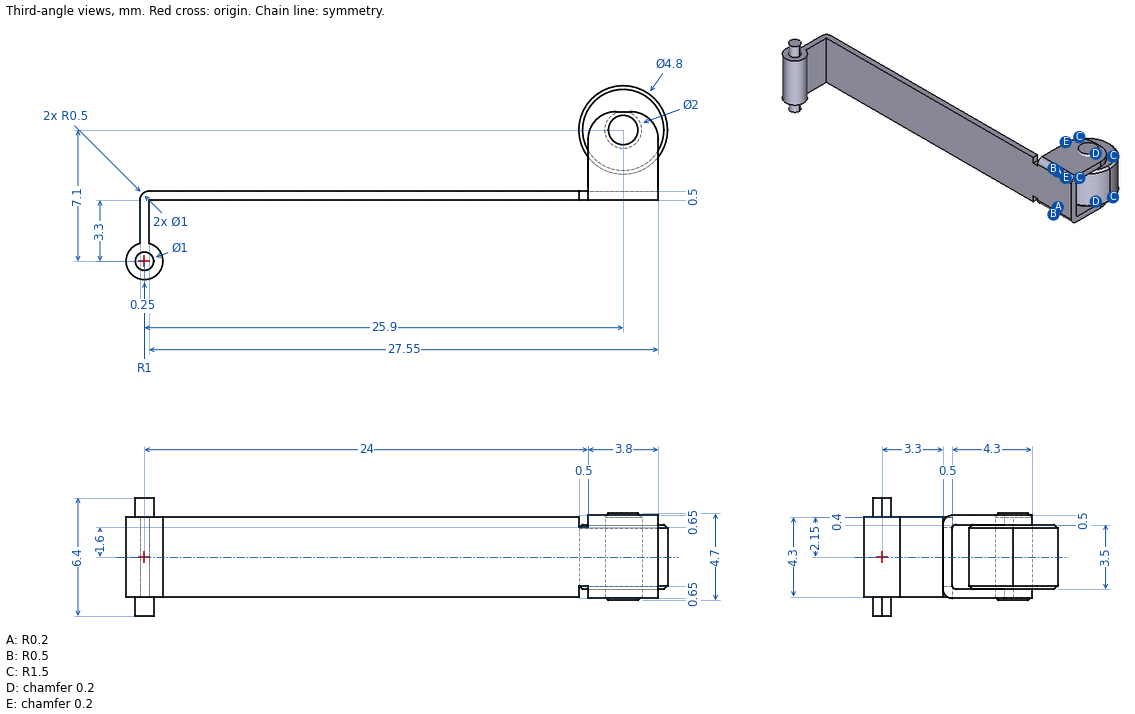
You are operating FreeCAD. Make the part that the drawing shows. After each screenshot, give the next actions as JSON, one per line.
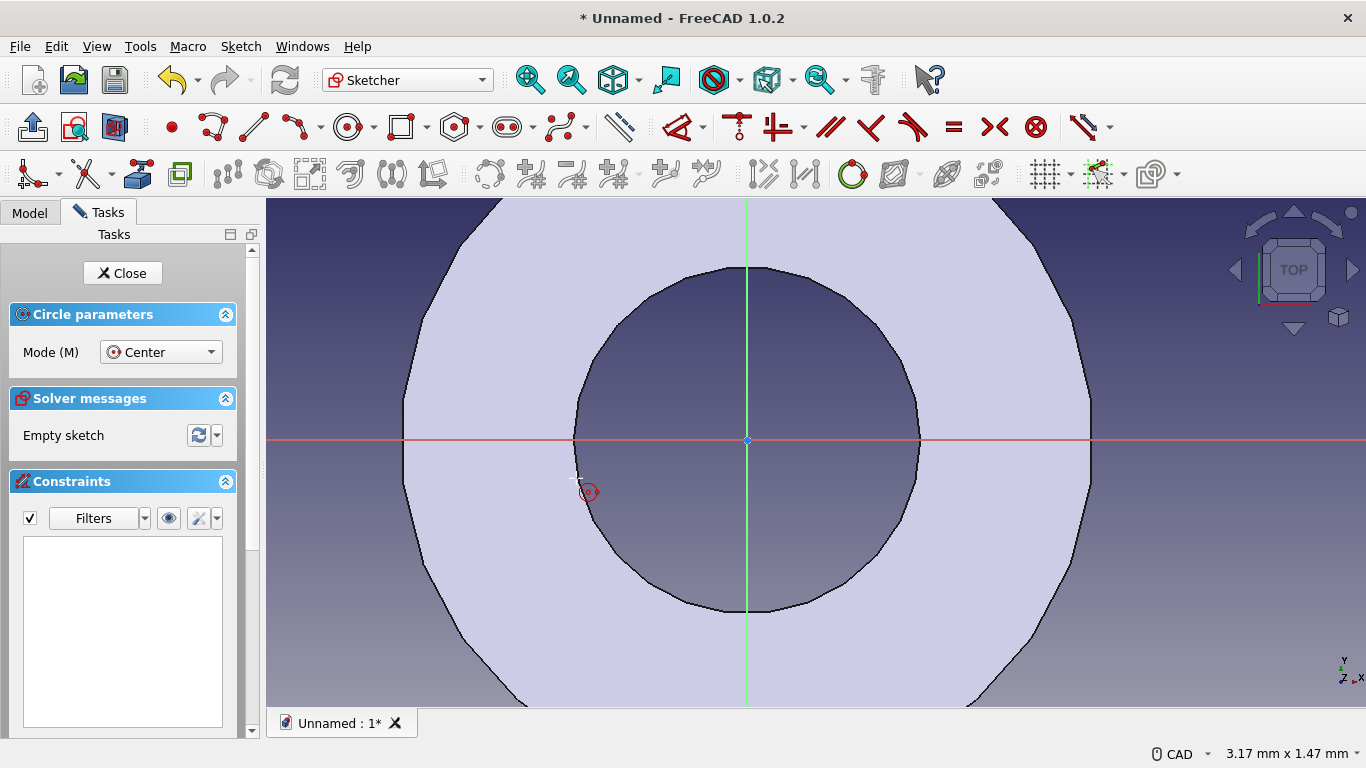
{"action": "left_click", "coordinate": [747, 440]}
{"action": "mouse_move", "coordinate": [870, 318]}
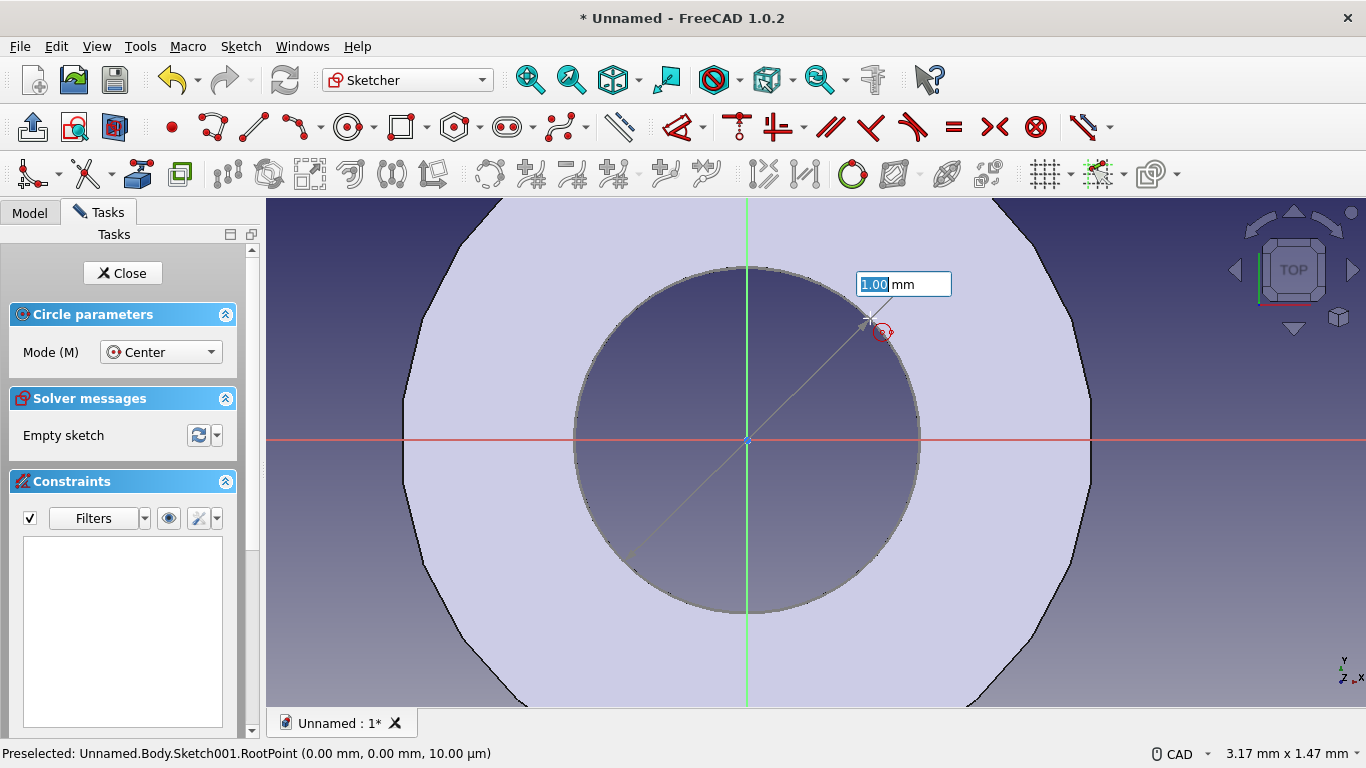
{"action": "type", "text": "1"}
{"action": "key", "text": "Return"}
{"action": "key", "text": "Escape"}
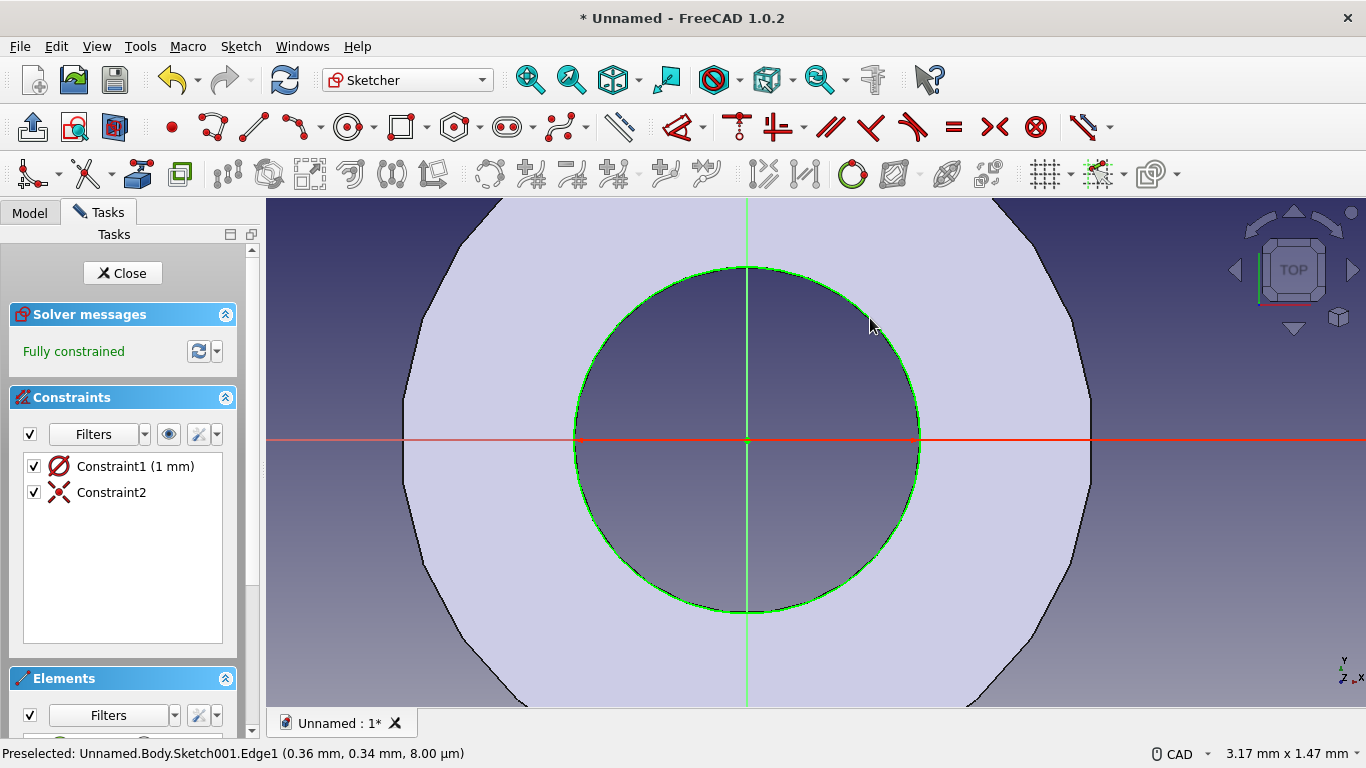
{"action": "left_click", "coordinate": [123, 273]}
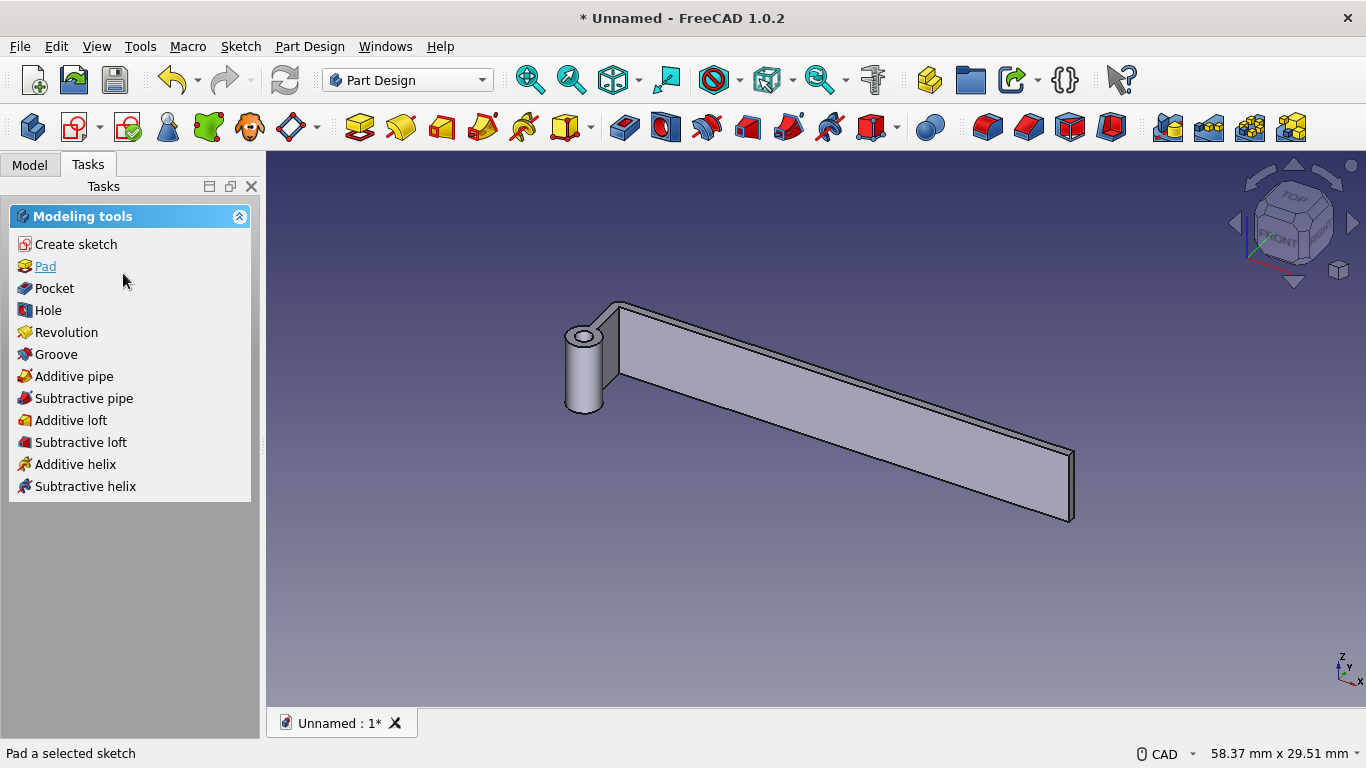
{"action": "left_click", "coordinate": [360, 128]}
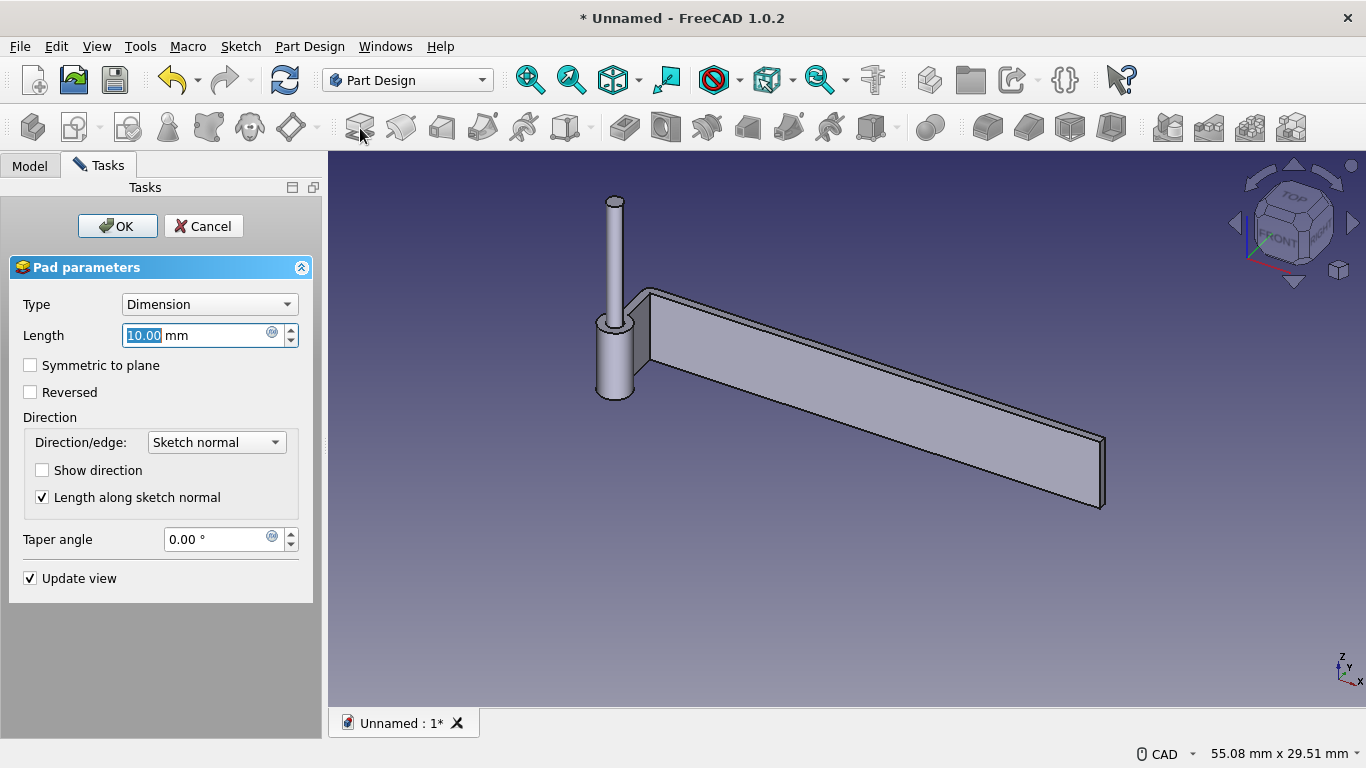
{"action": "type", "text": "6.4"}
{"action": "key", "text": "Tab"}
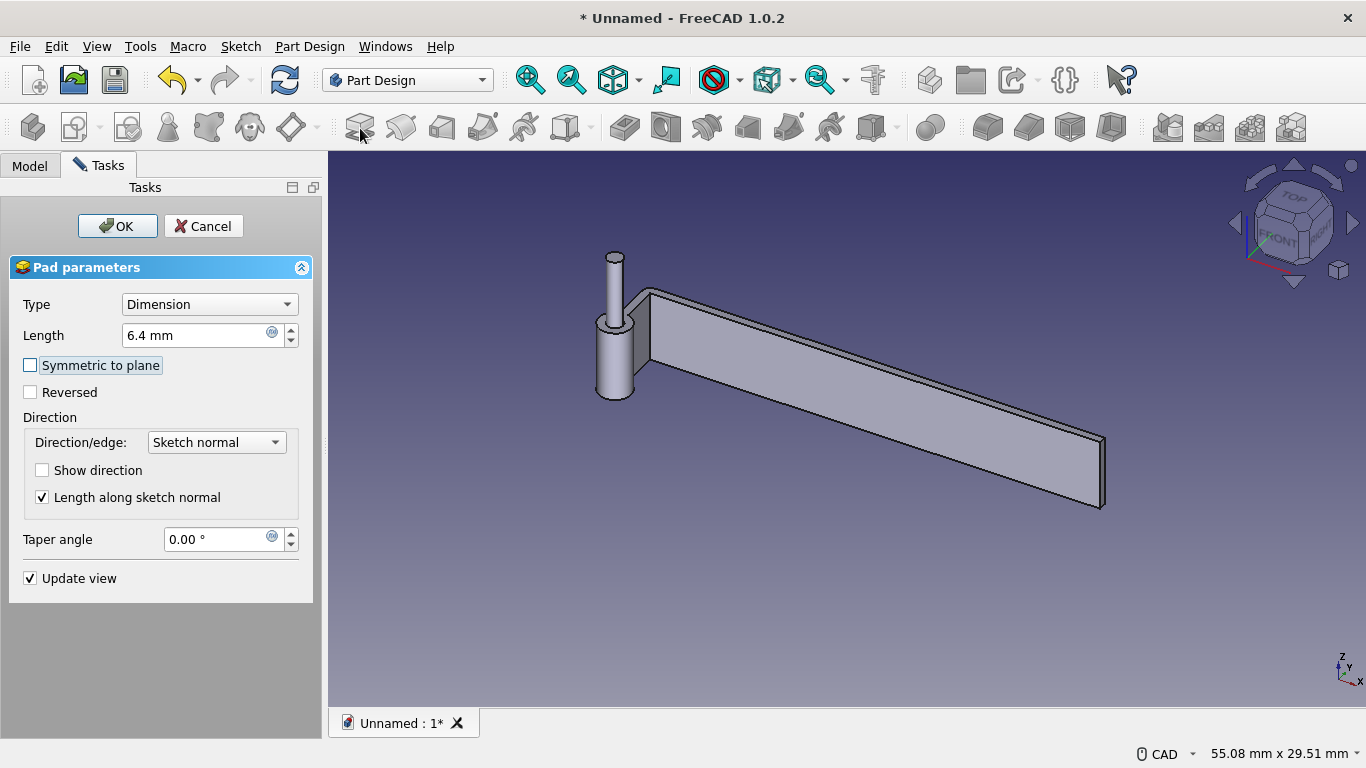
{"action": "left_click", "coordinate": [31, 365]}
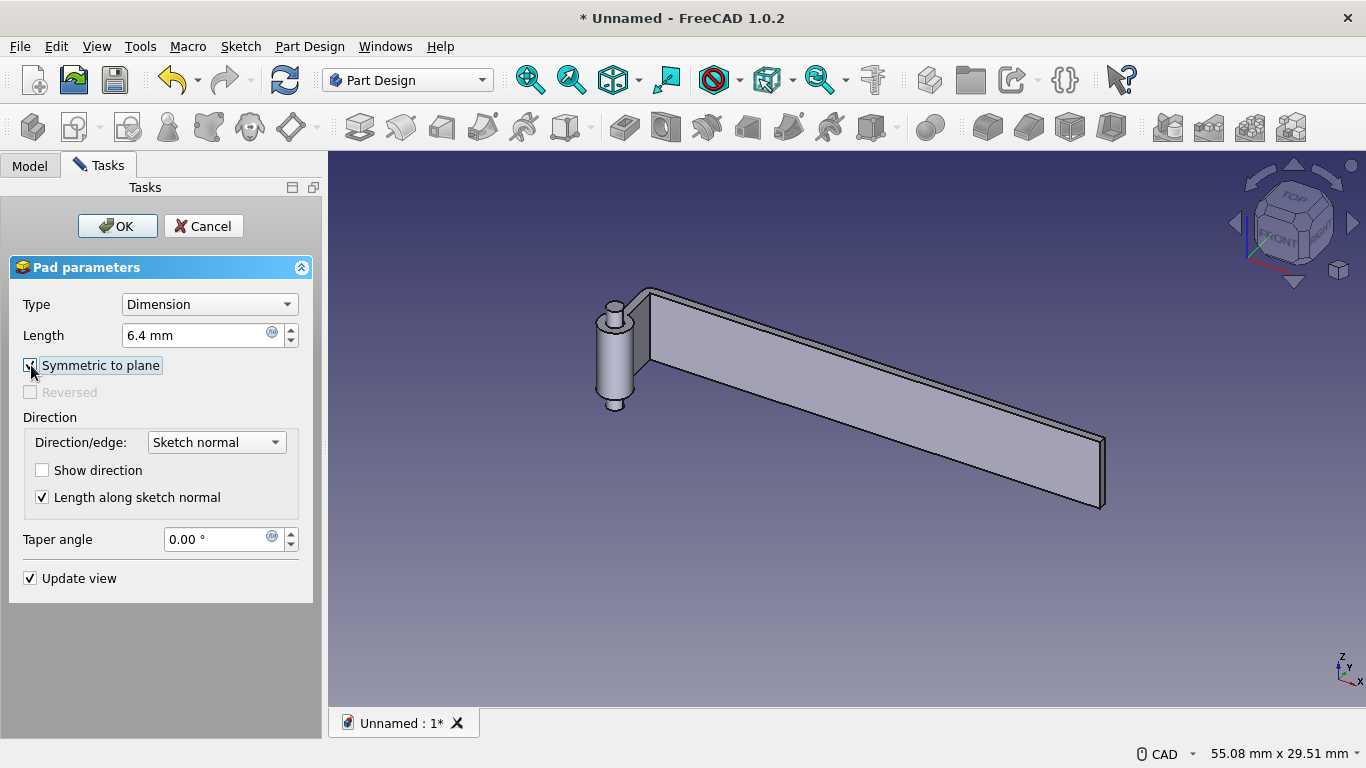
{"action": "left_click", "coordinate": [118, 226]}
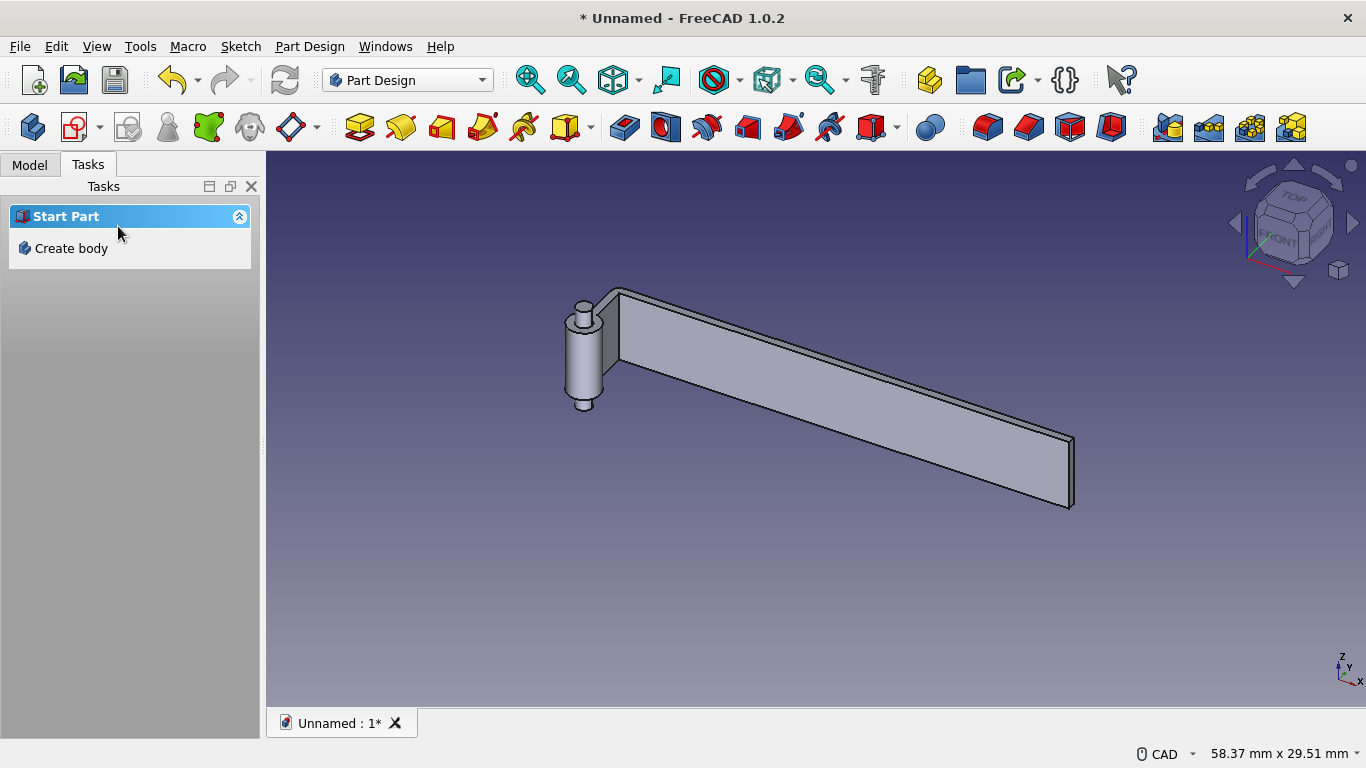
{"action": "scroll", "coordinate": [1071, 444], "scroll_direction": "up", "scroll_amount": 5}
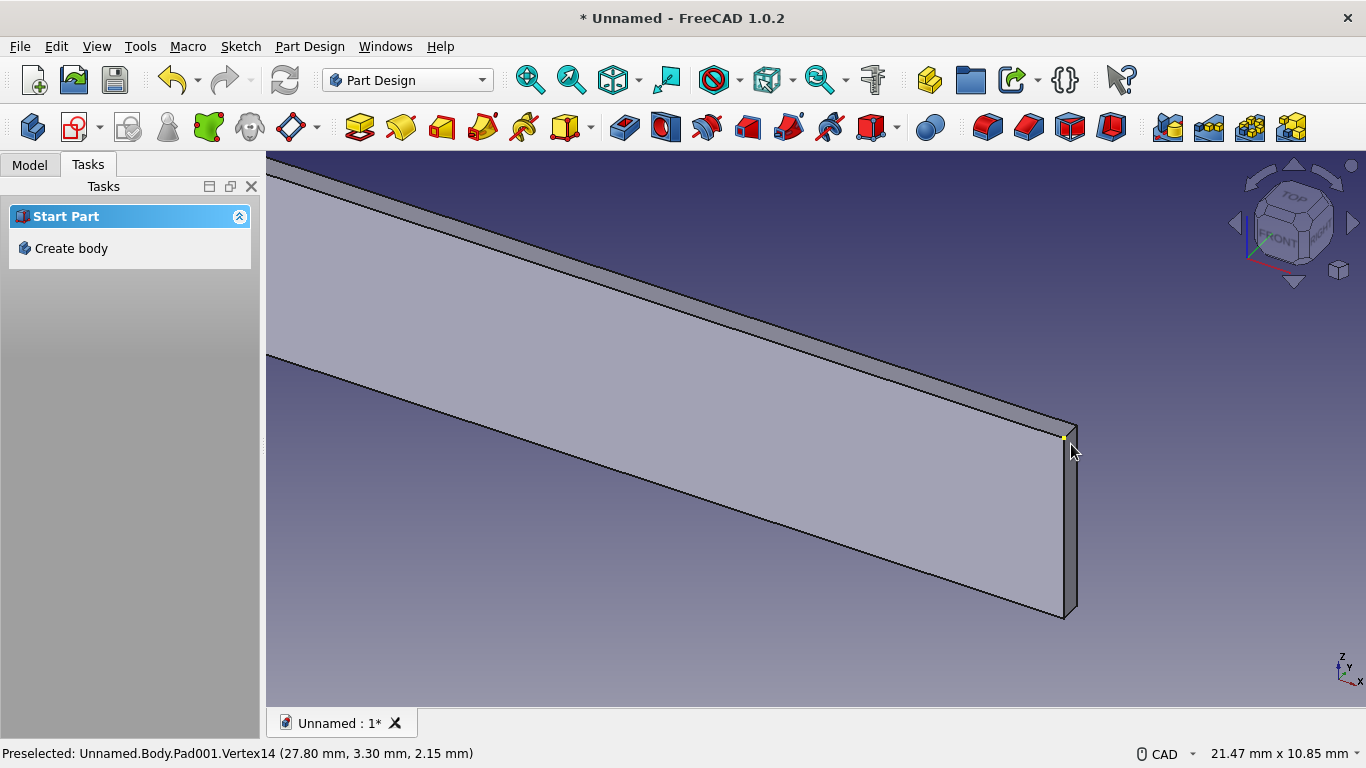
{"action": "key", "text": "v f"}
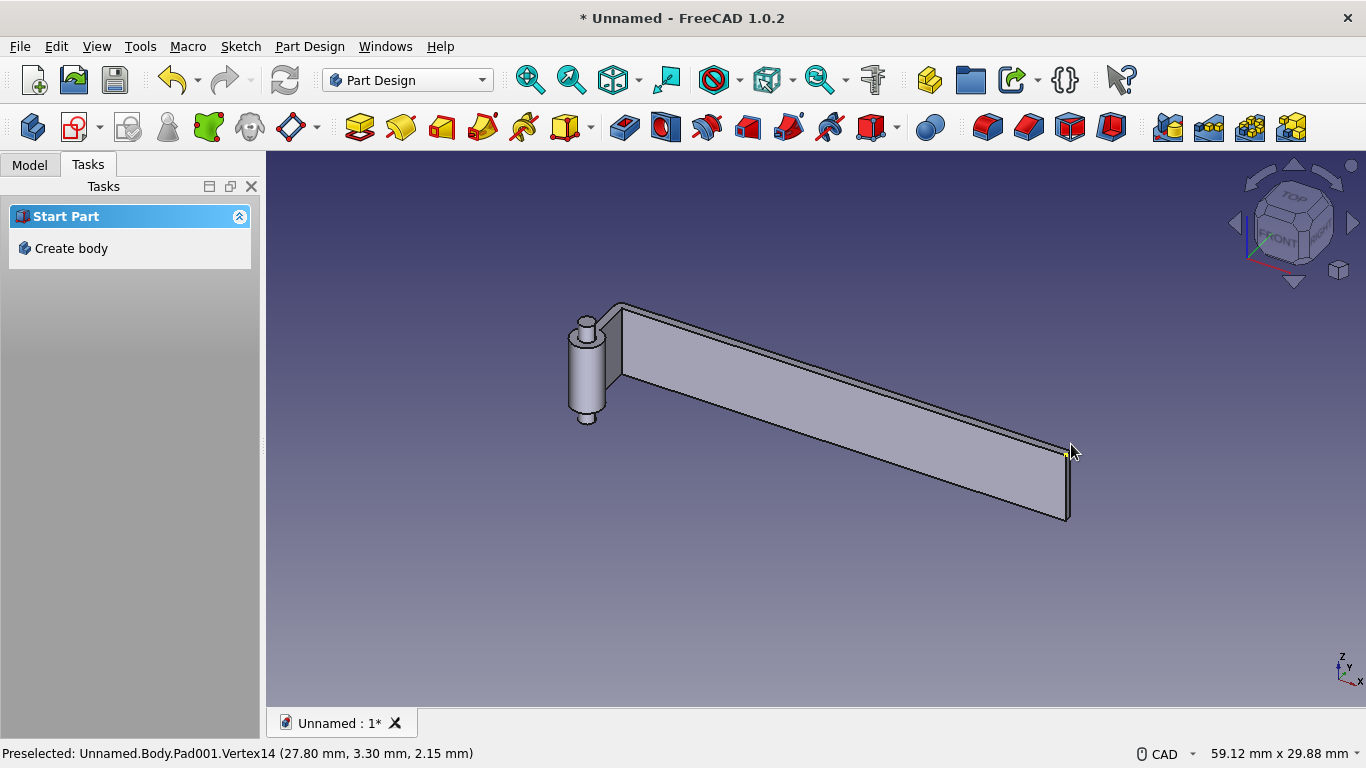
{"action": "key", "text": "0"}